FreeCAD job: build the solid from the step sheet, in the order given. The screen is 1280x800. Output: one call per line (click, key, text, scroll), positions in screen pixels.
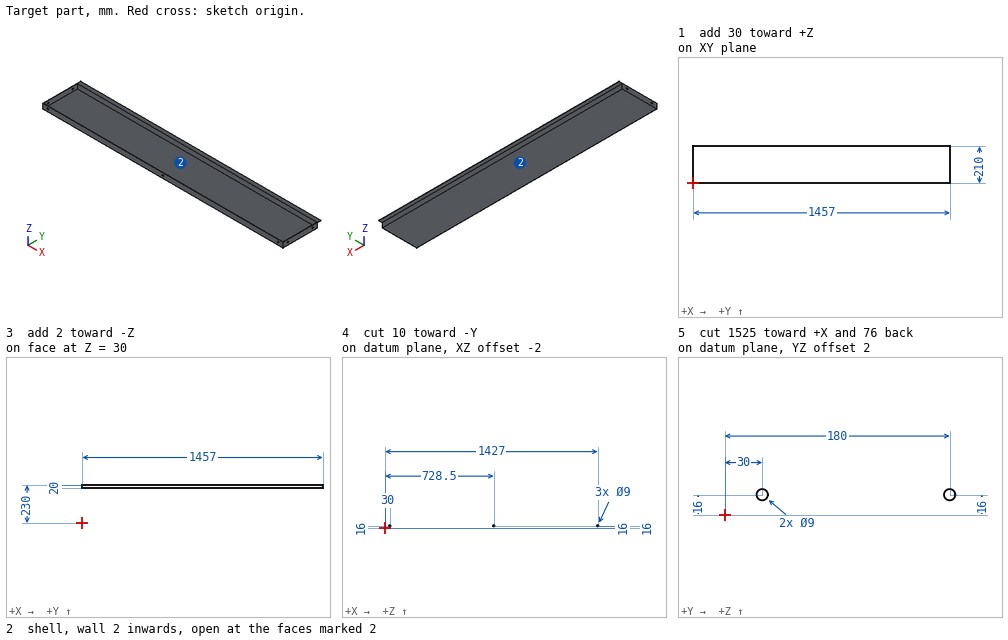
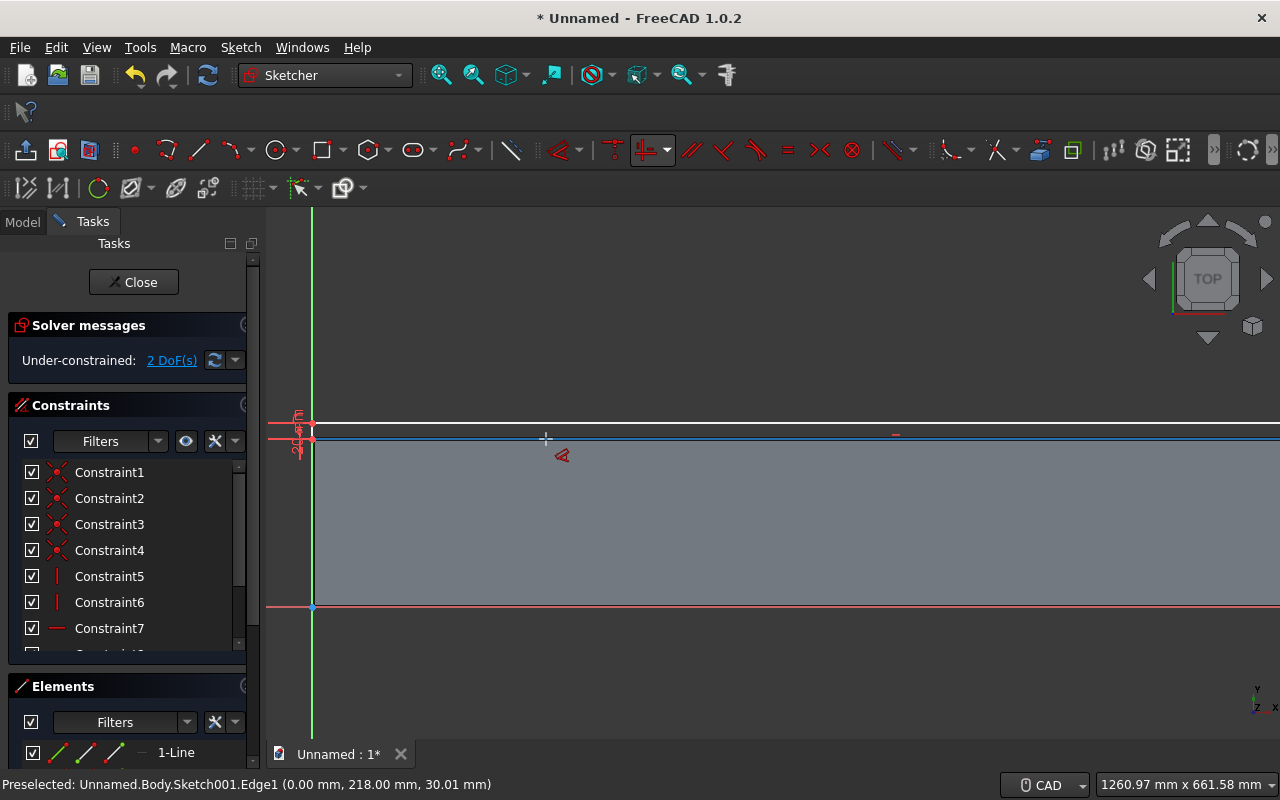
click(547, 439)
click(714, 405)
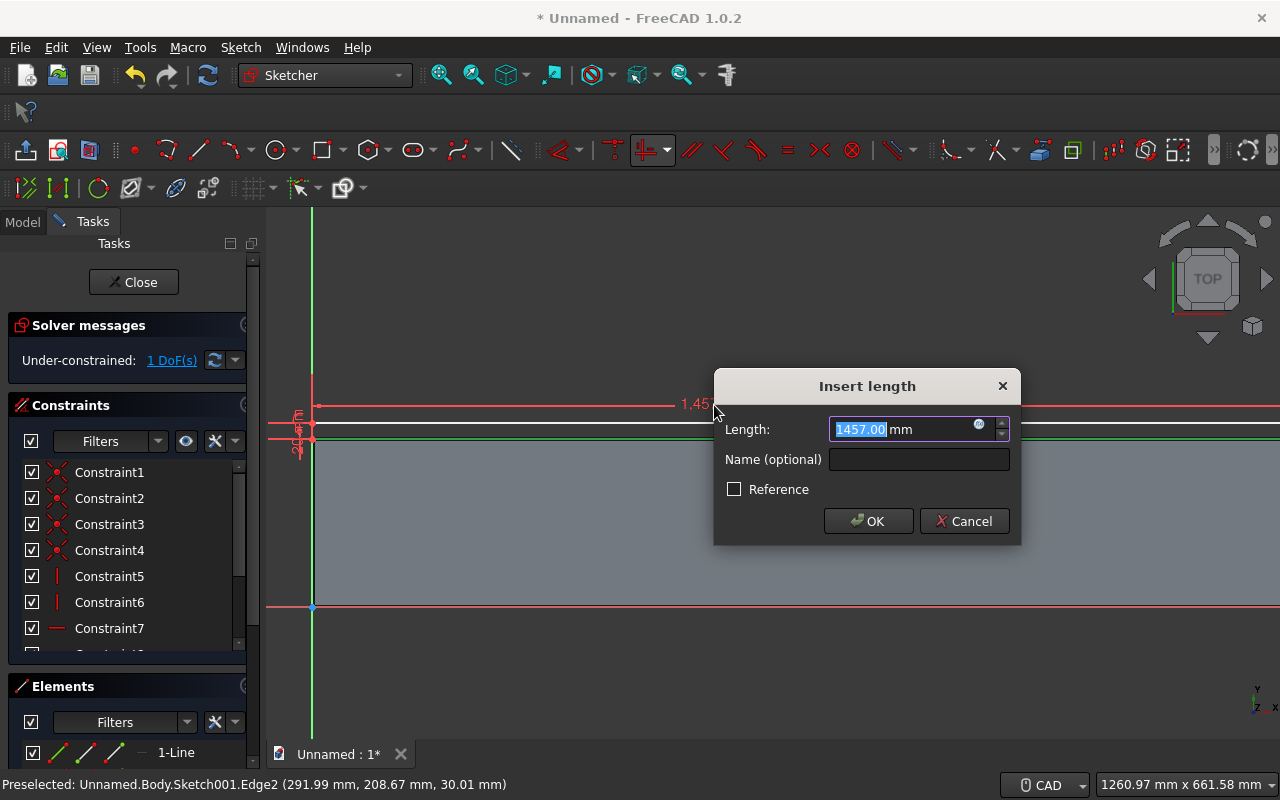
text(1457)
key(Return)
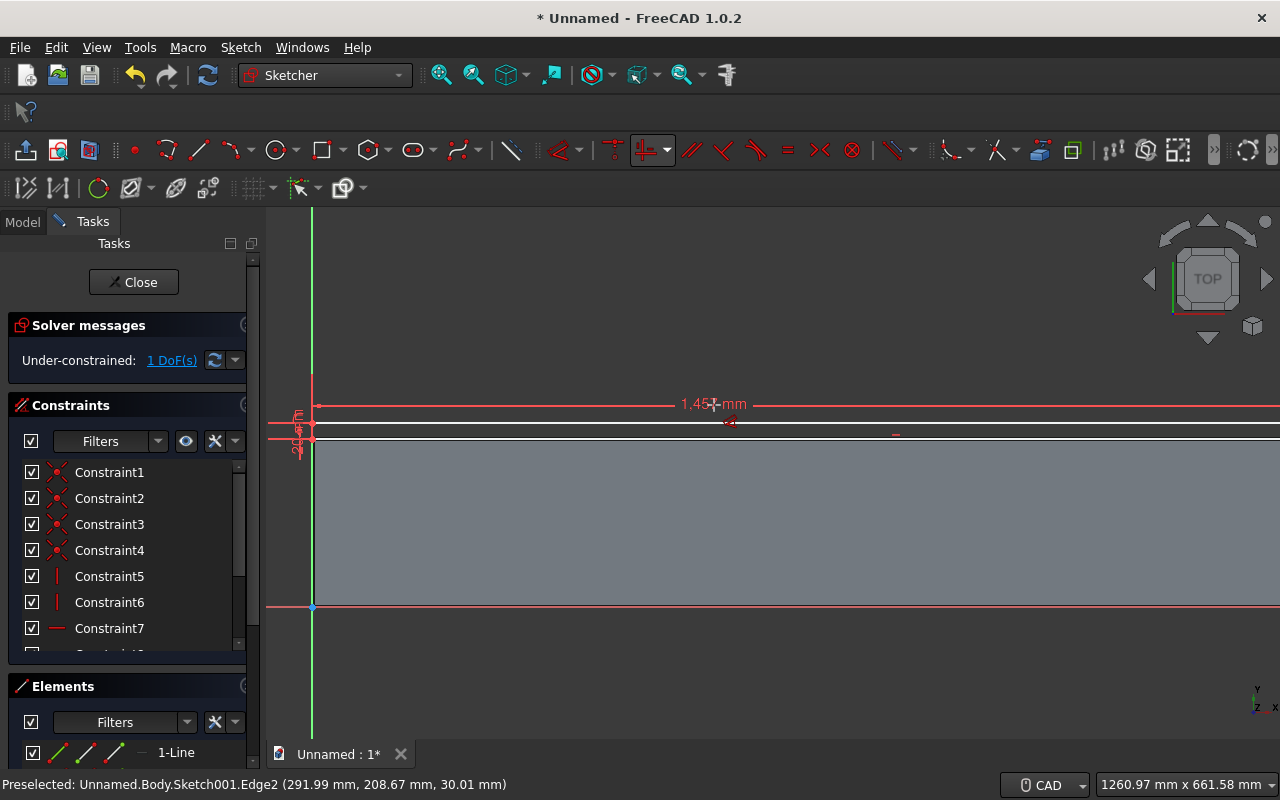
click(312, 423)
click(346, 515)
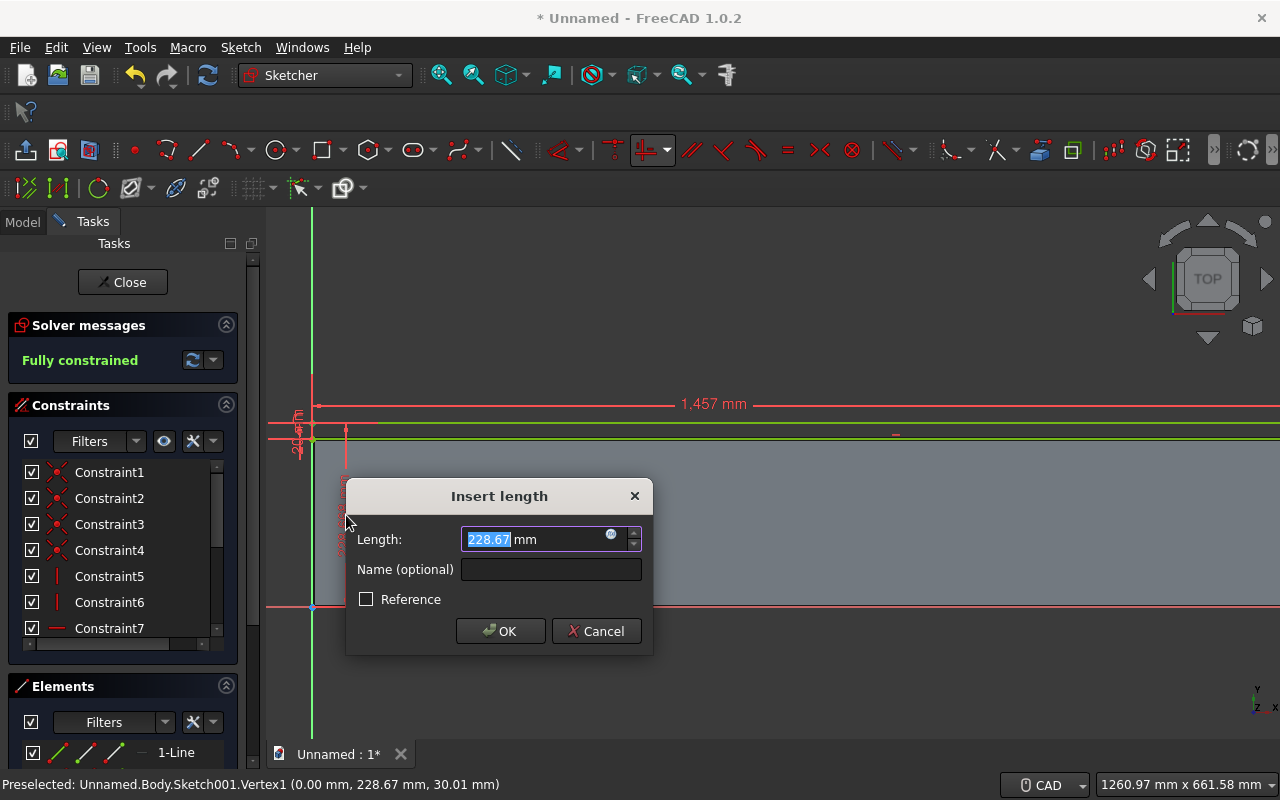
text(230)
key(Return)
key(Escape)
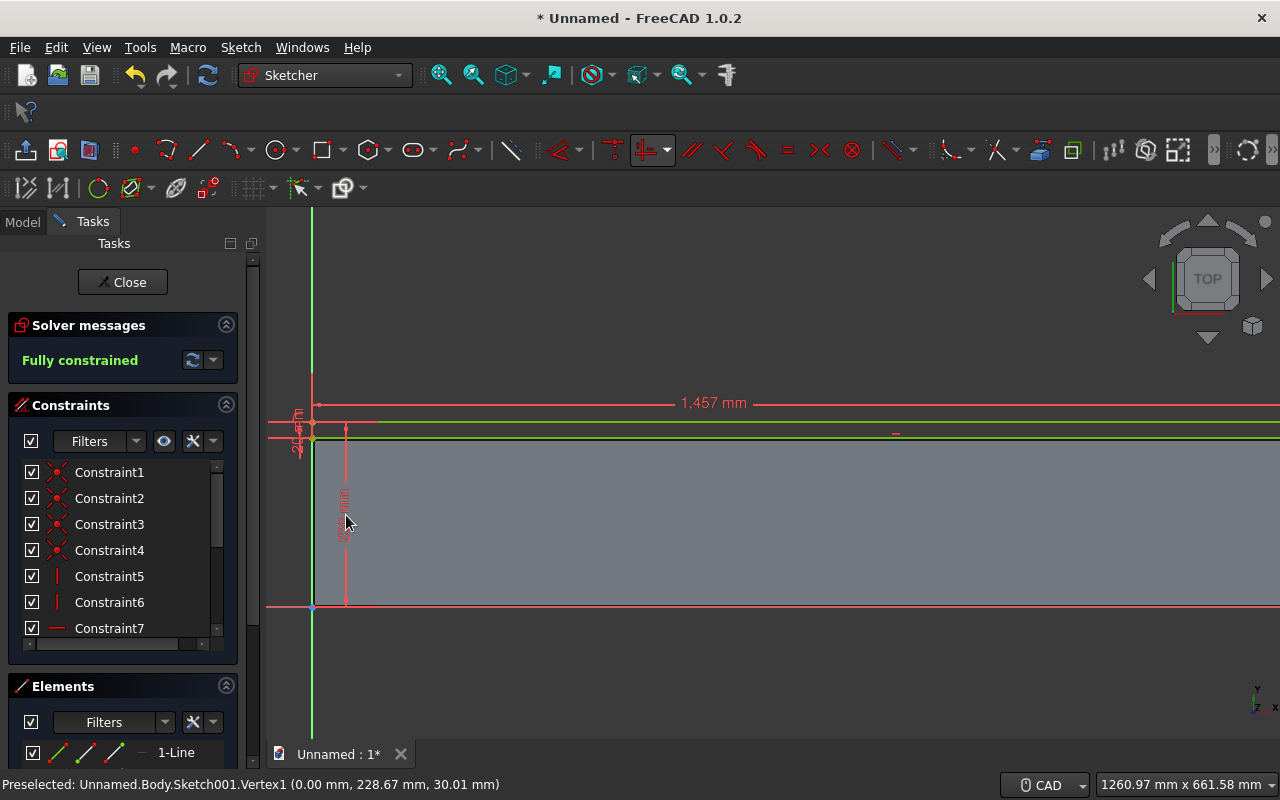
click(123, 282)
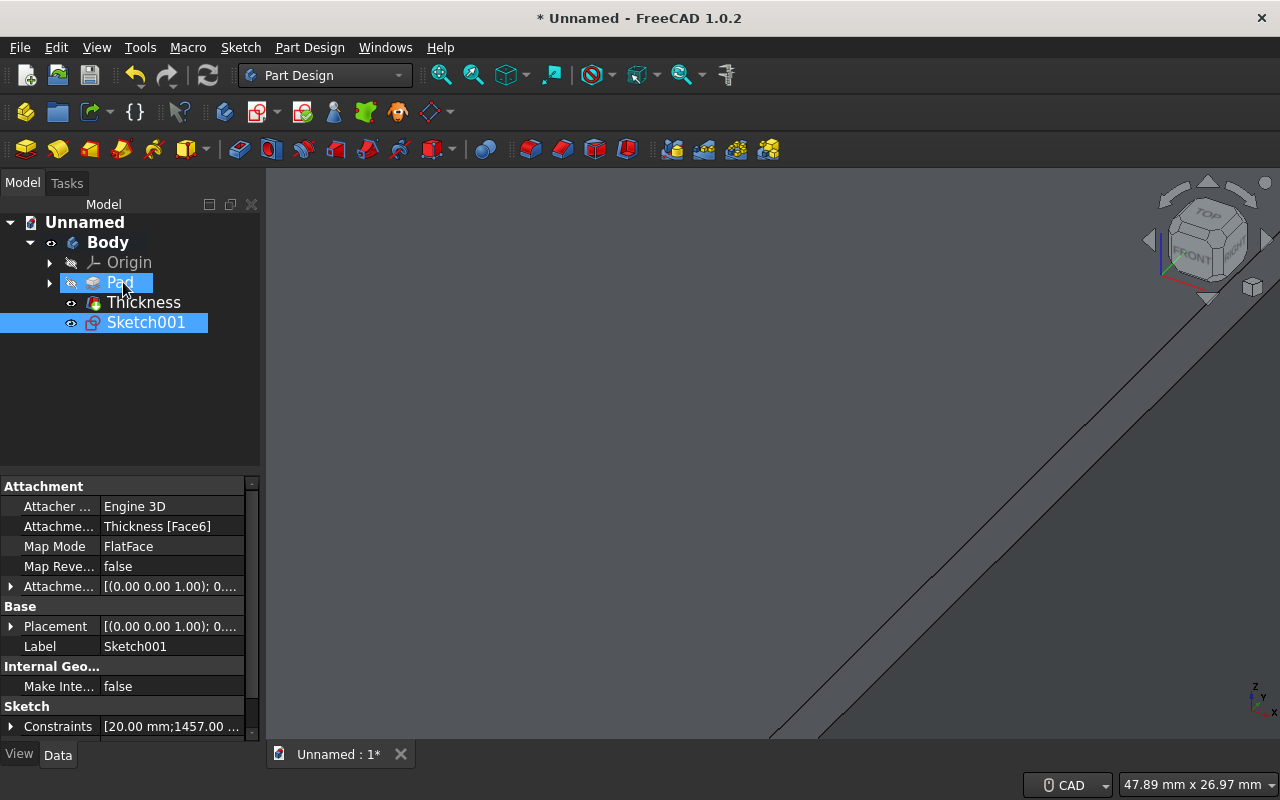
click(26, 150)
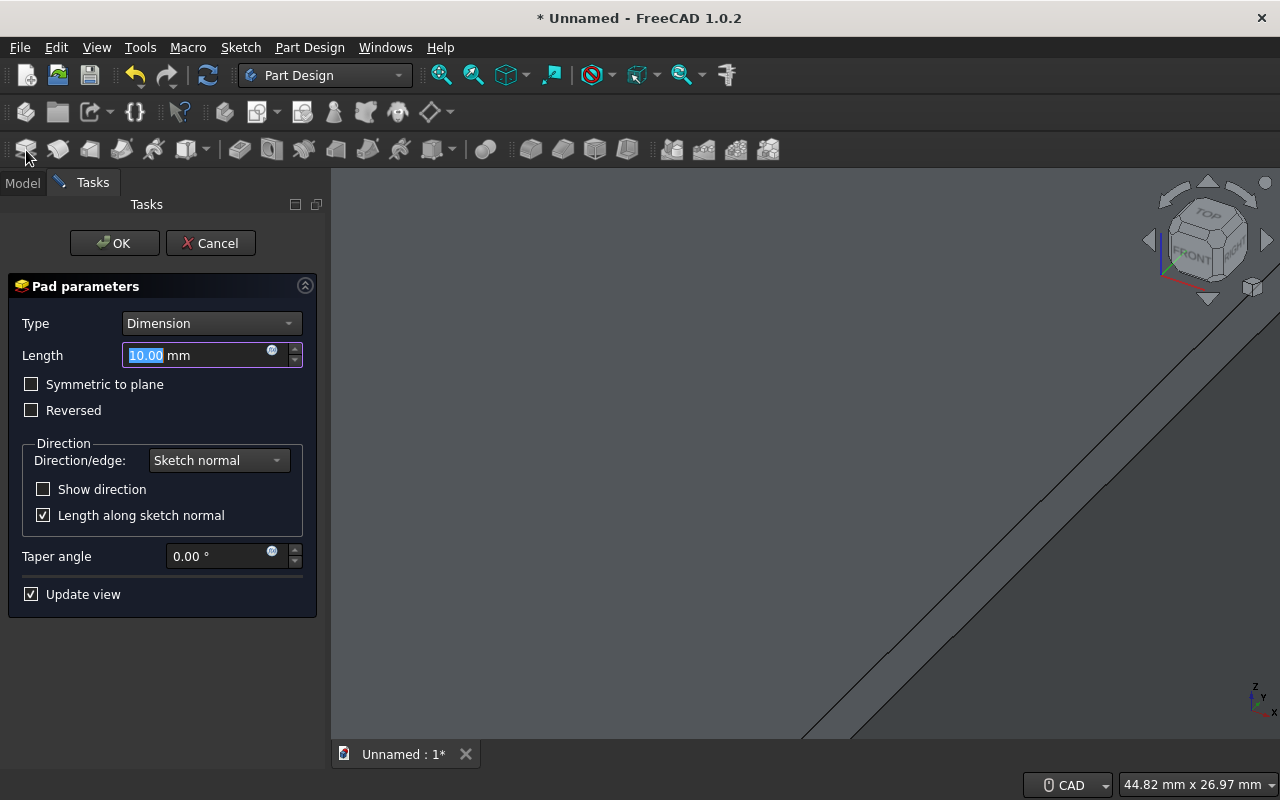
text(2)
key(Tab)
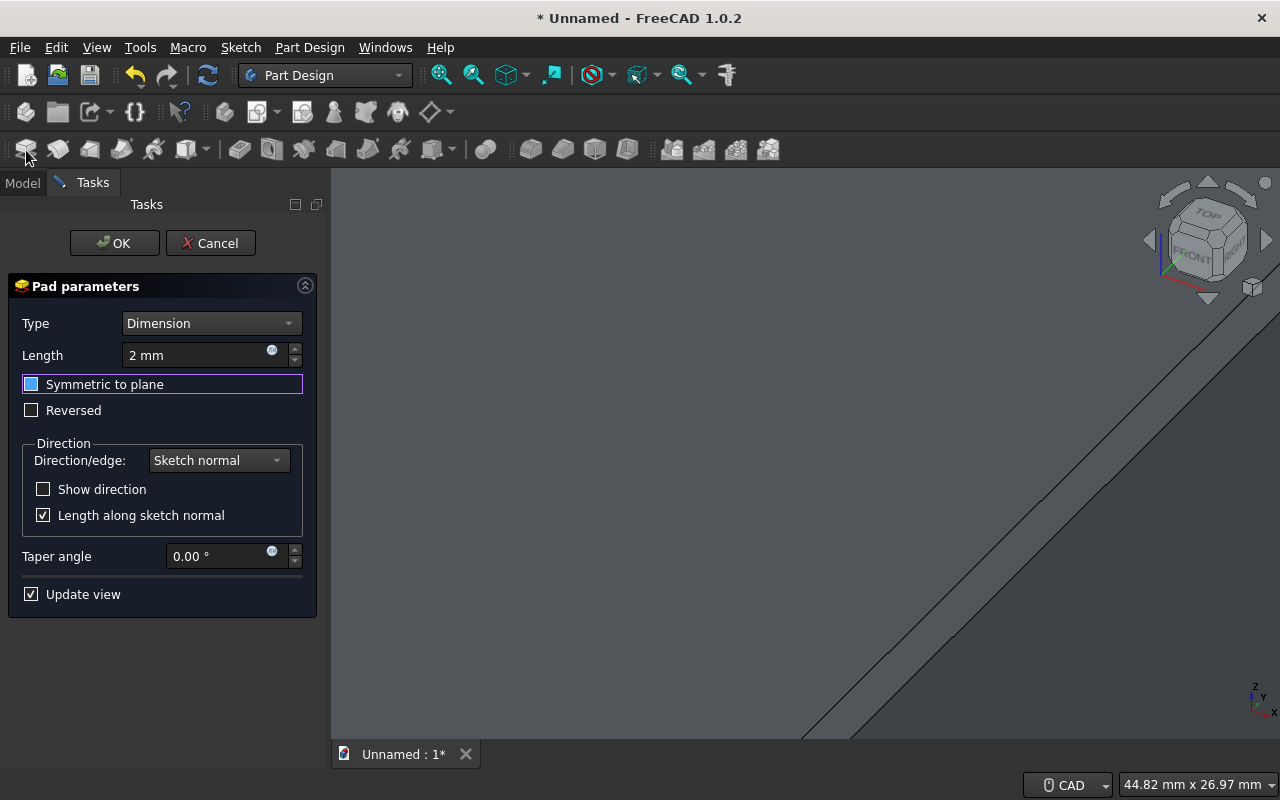
click(30, 410)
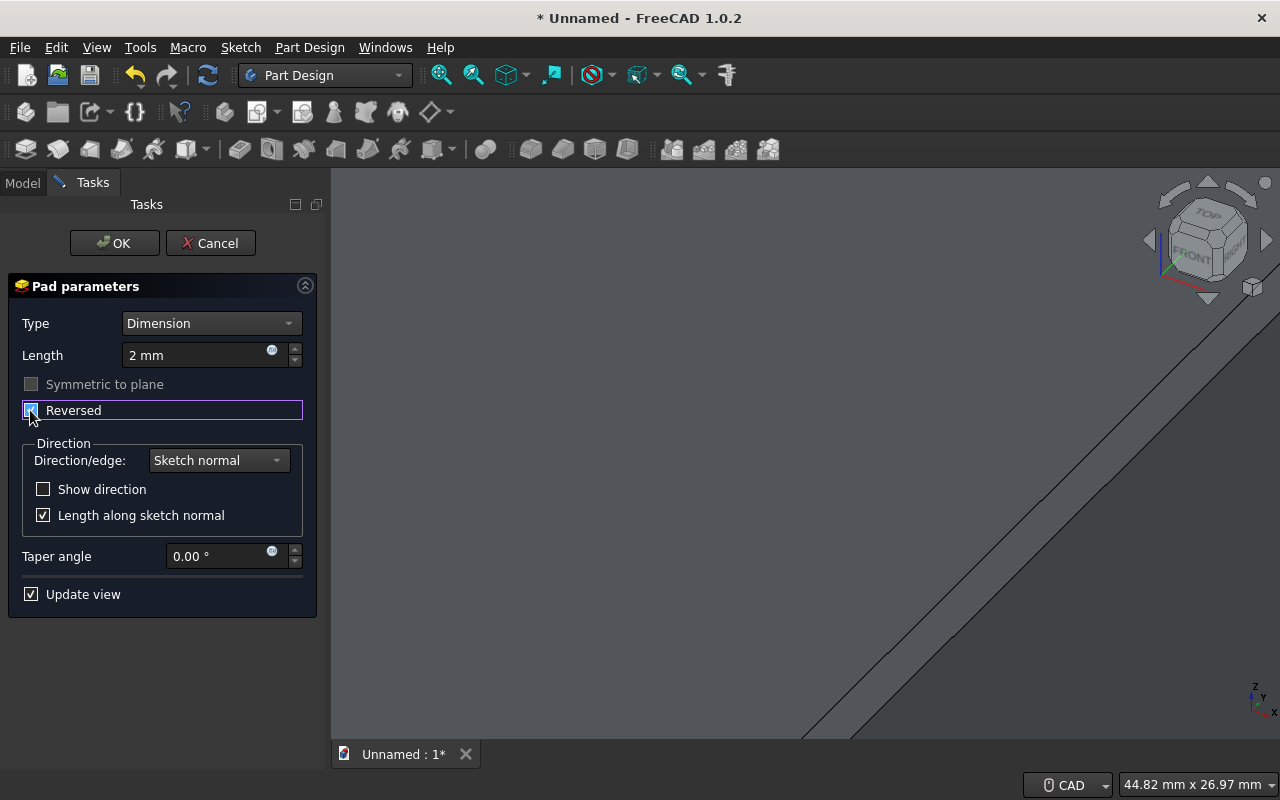
click(115, 243)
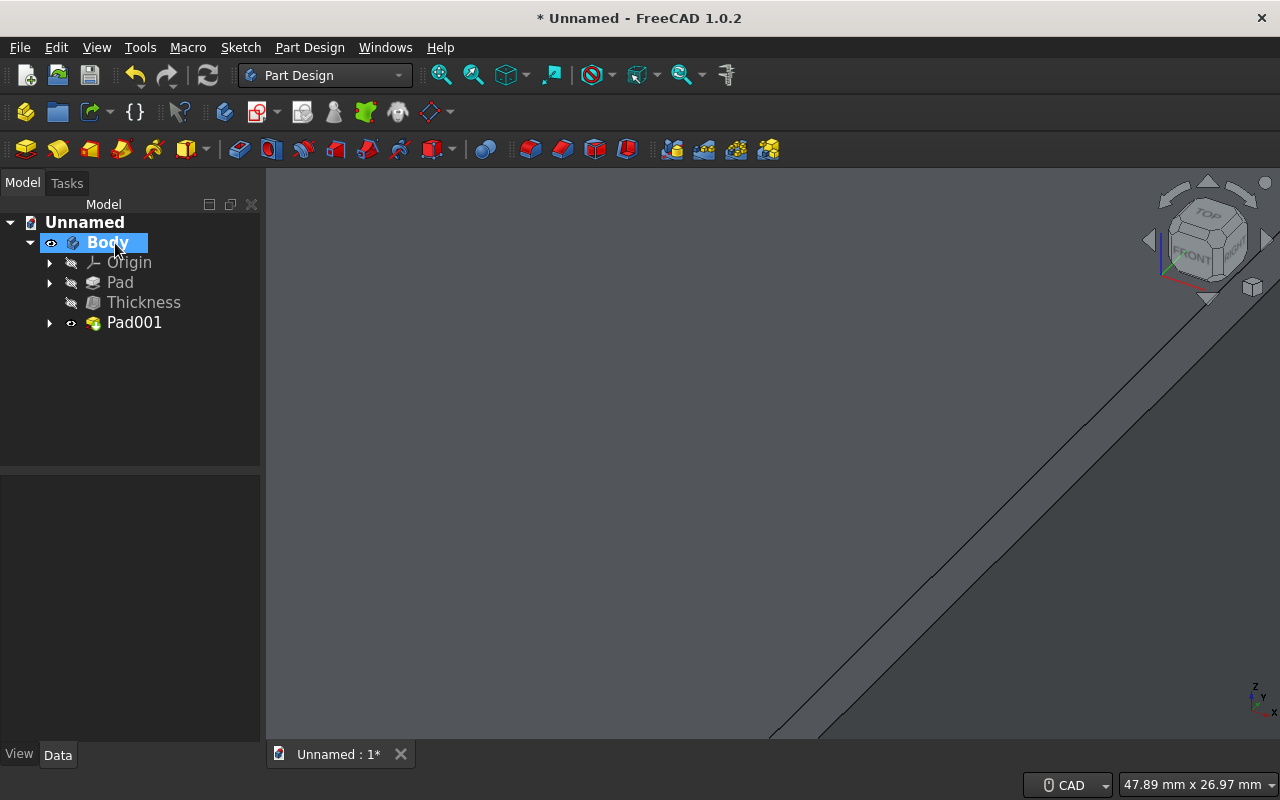
click(442, 76)